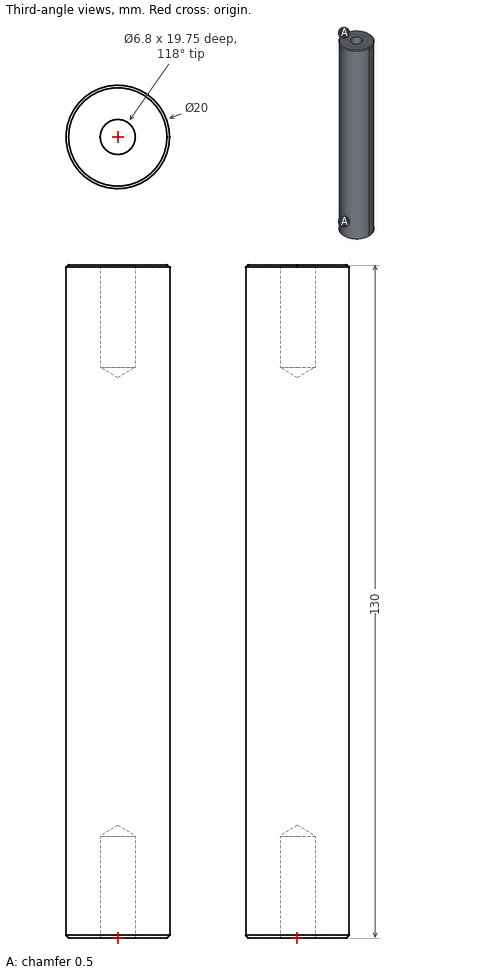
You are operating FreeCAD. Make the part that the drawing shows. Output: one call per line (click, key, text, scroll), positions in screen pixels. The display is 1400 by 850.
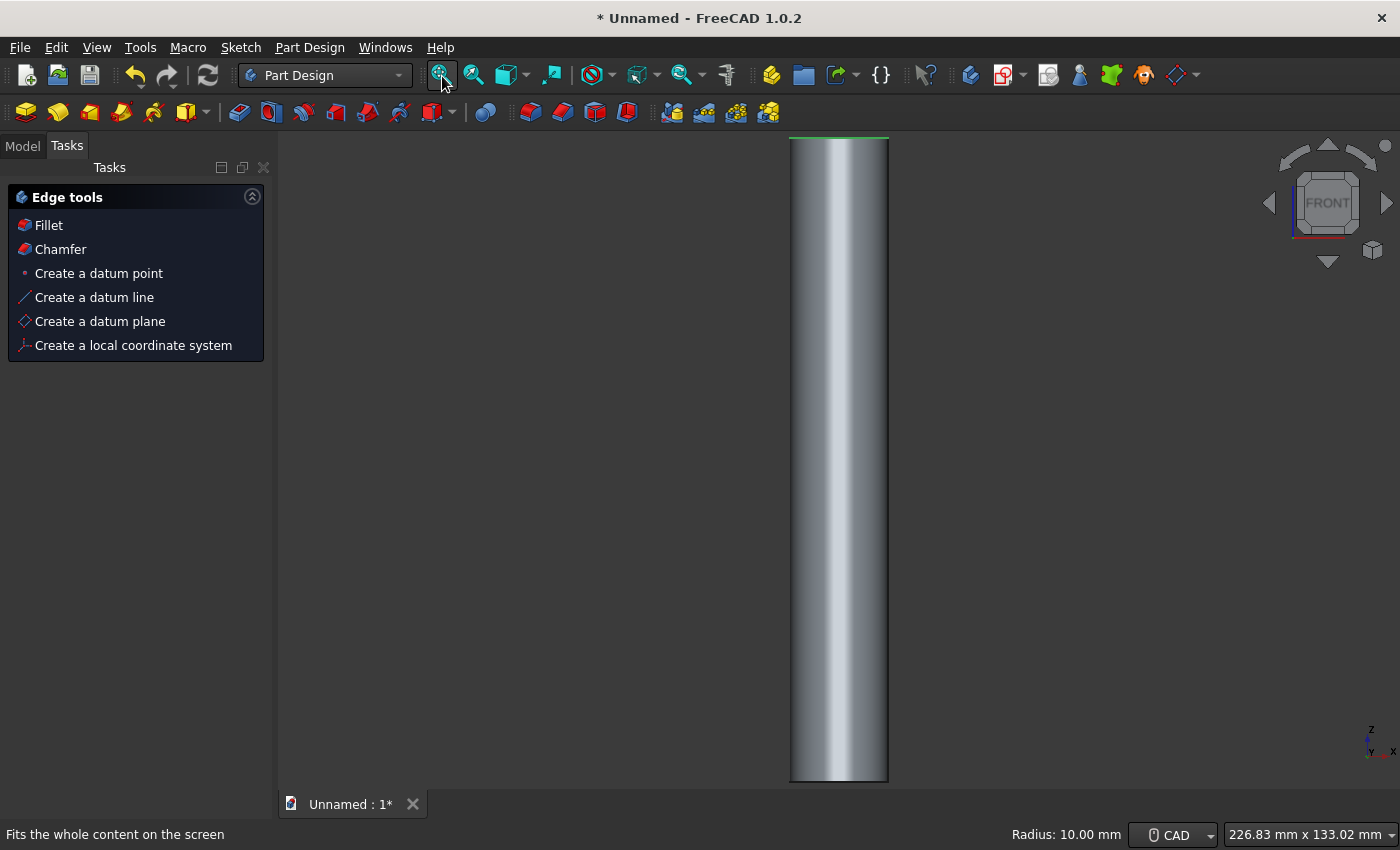
key(3)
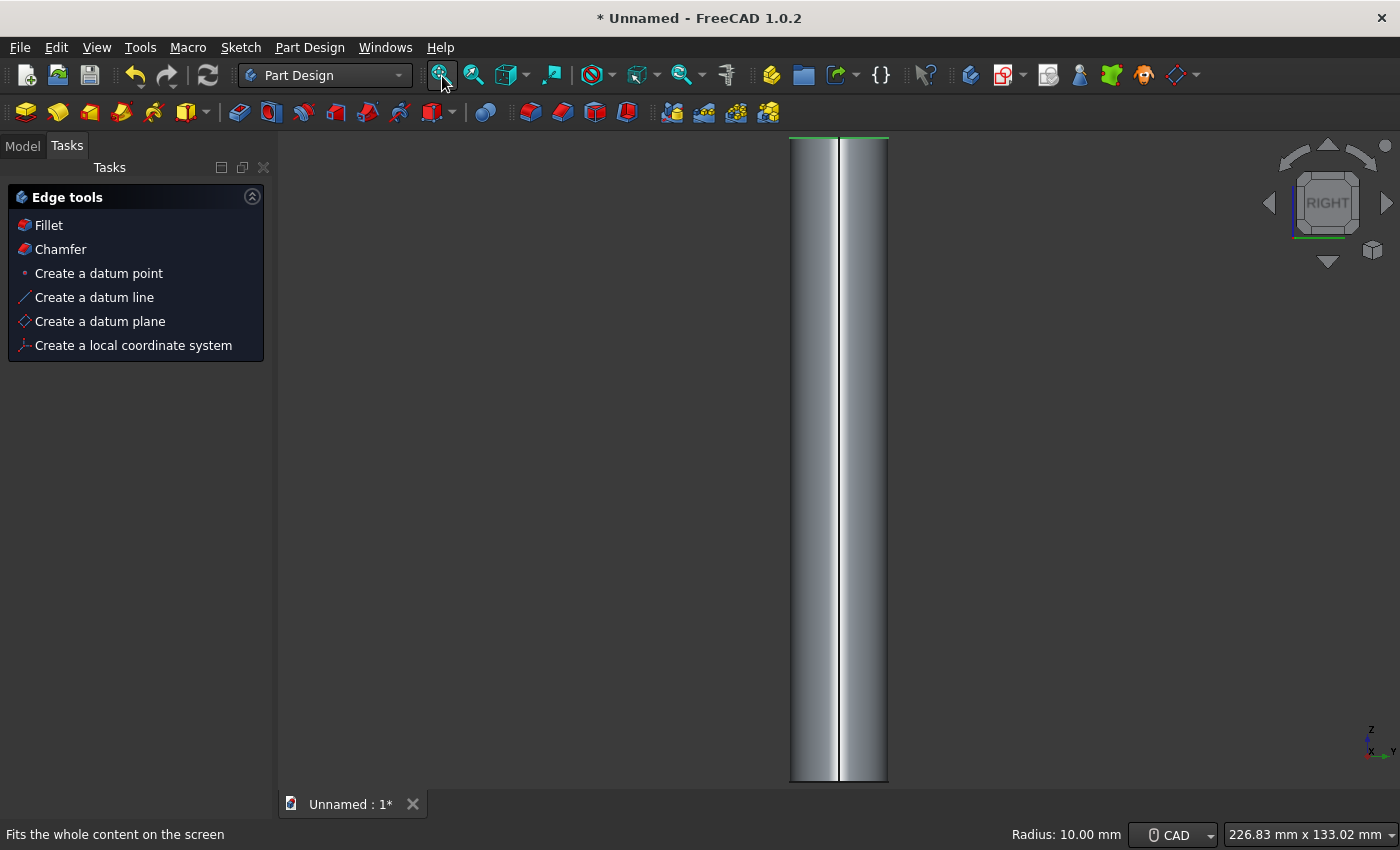
key(5)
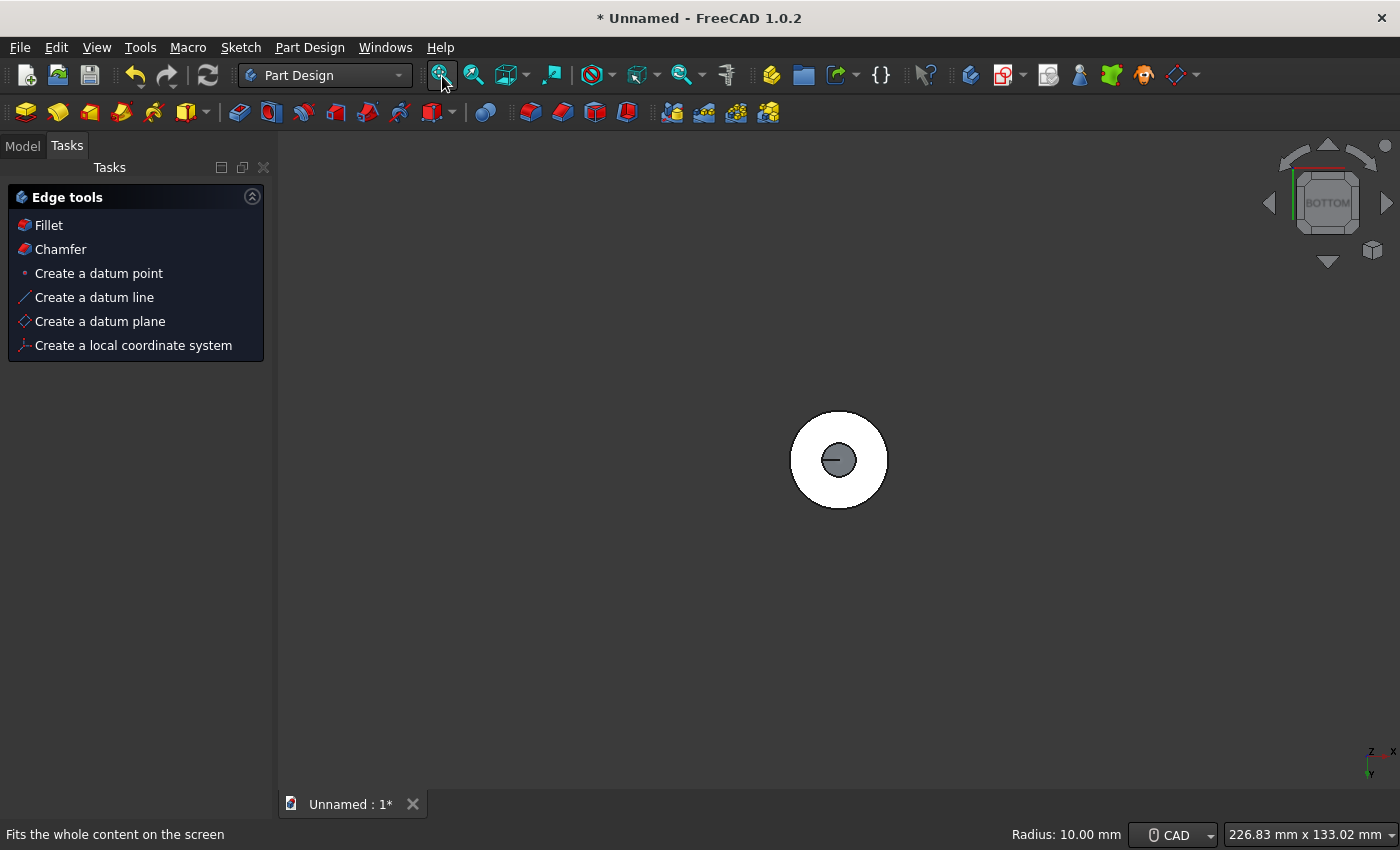
key(v)
key(f)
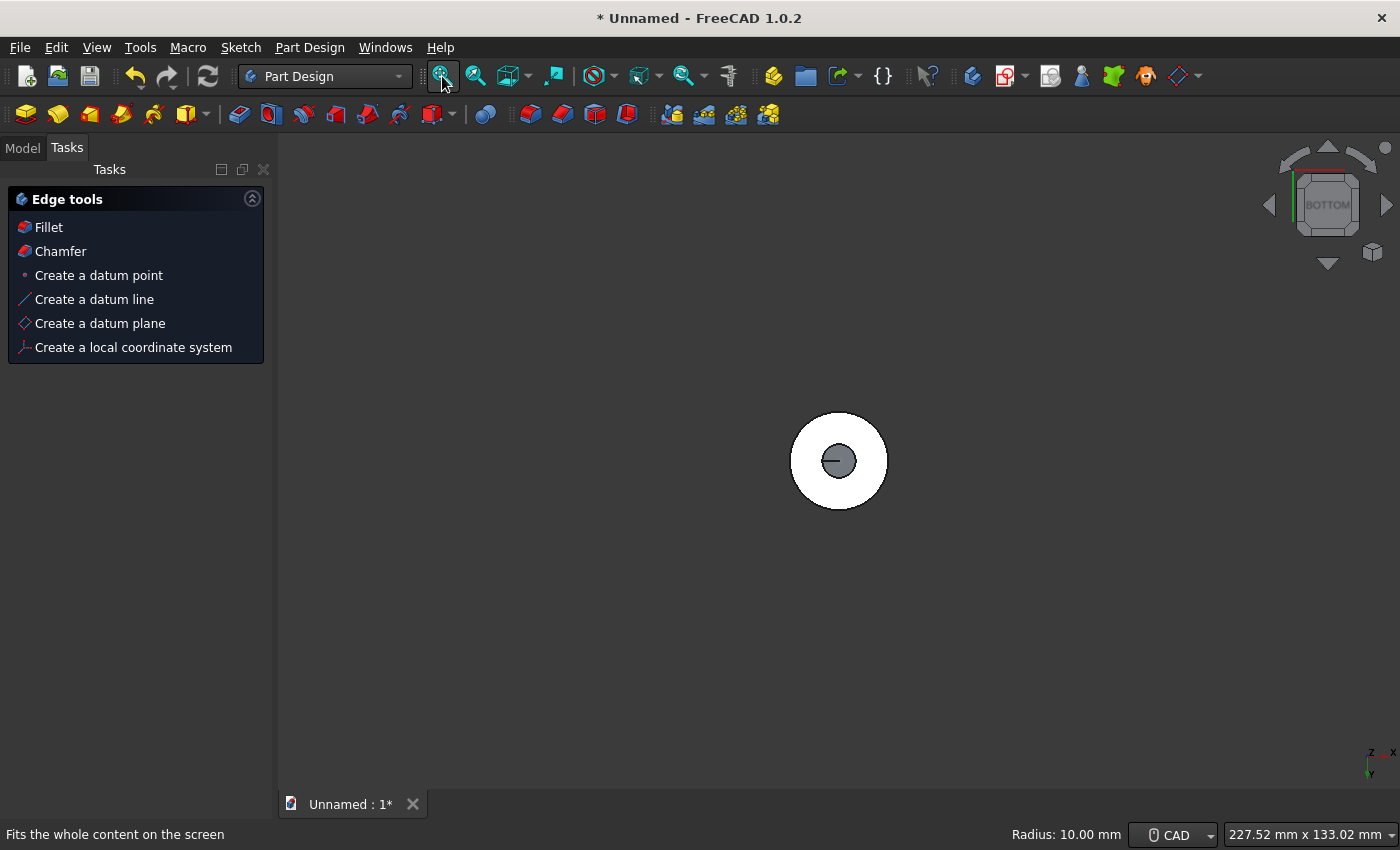
click(790, 460, ctrl)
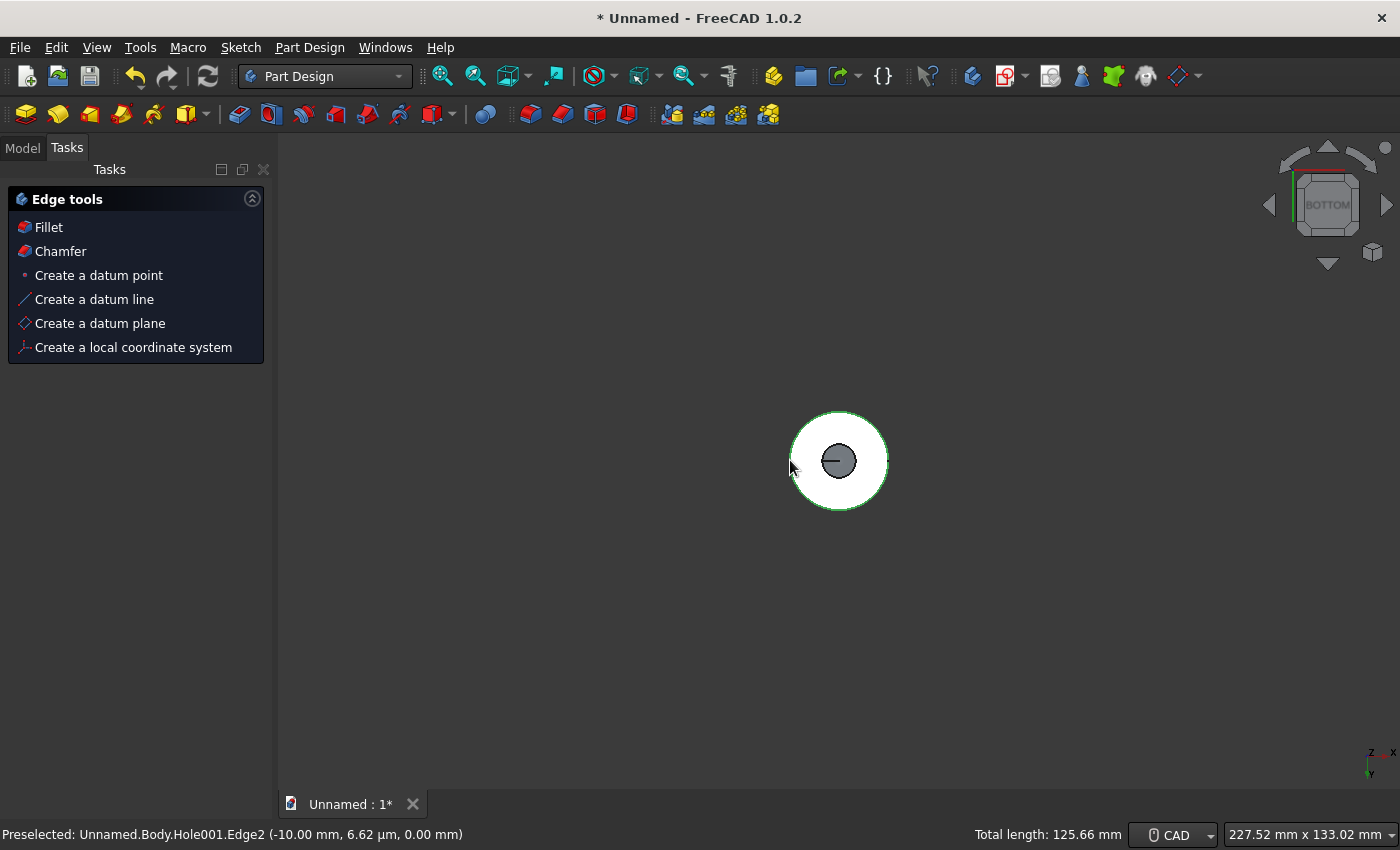
click(564, 114)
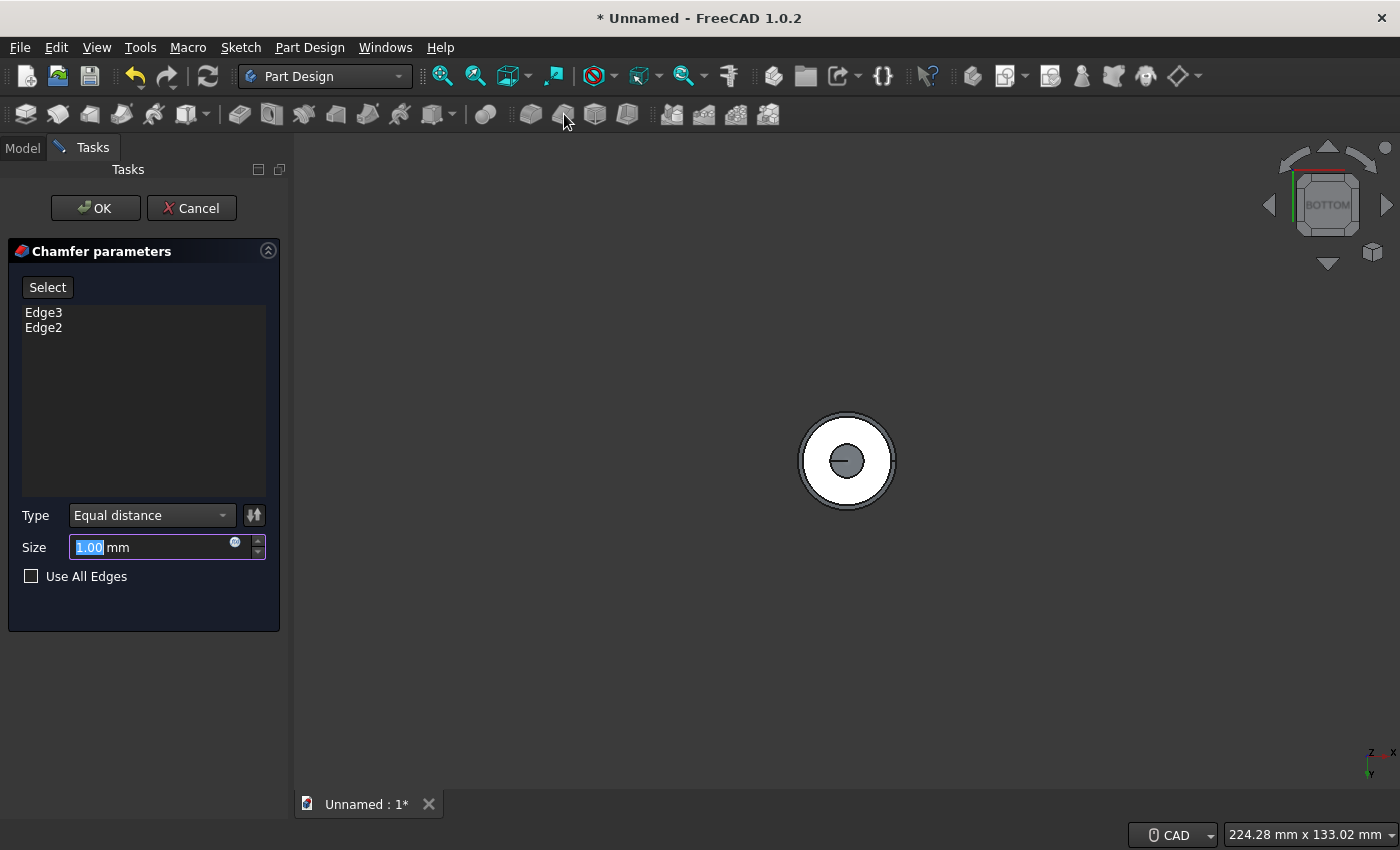
text(0.5)
key(Tab)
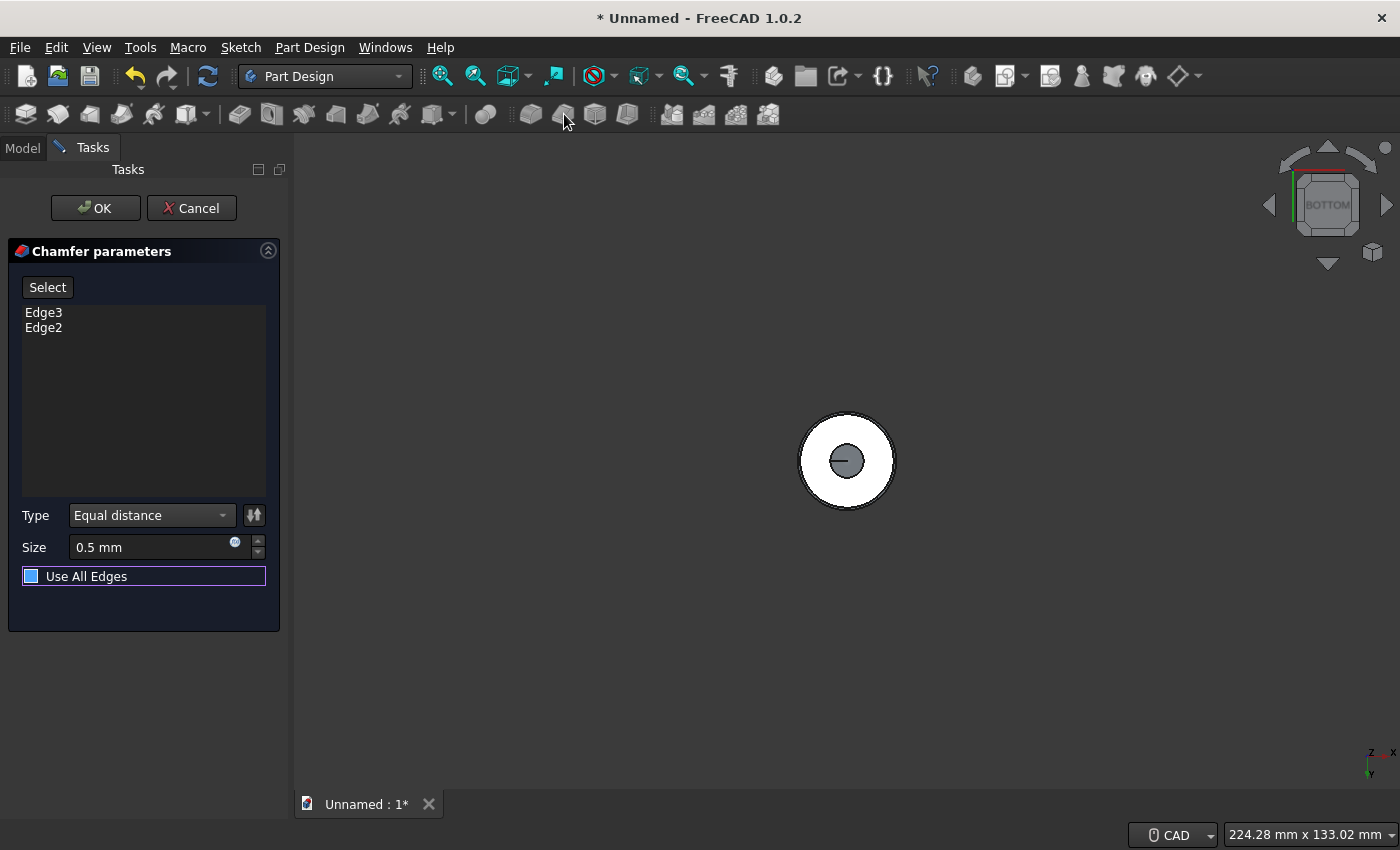
click(96, 208)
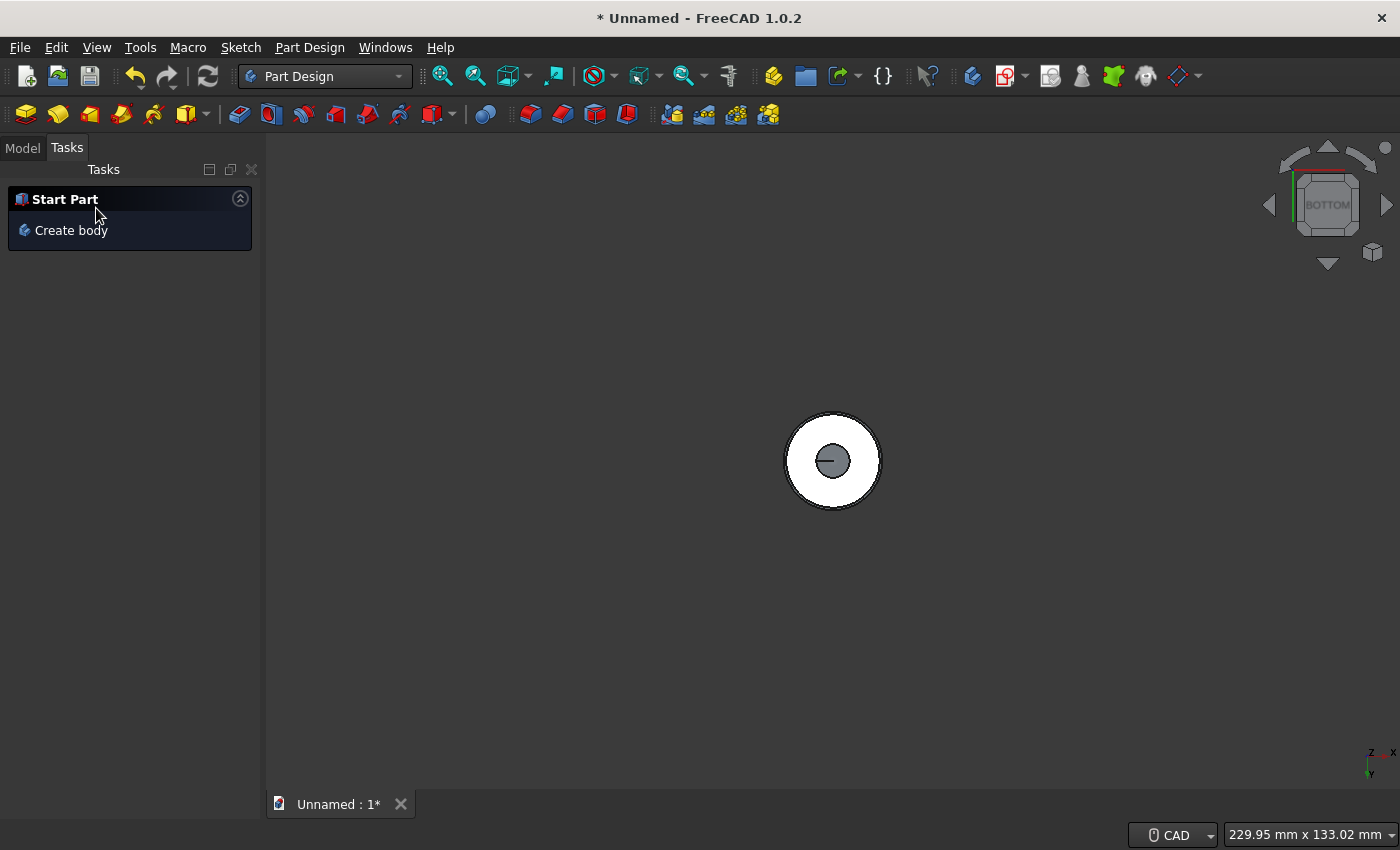
key(0)